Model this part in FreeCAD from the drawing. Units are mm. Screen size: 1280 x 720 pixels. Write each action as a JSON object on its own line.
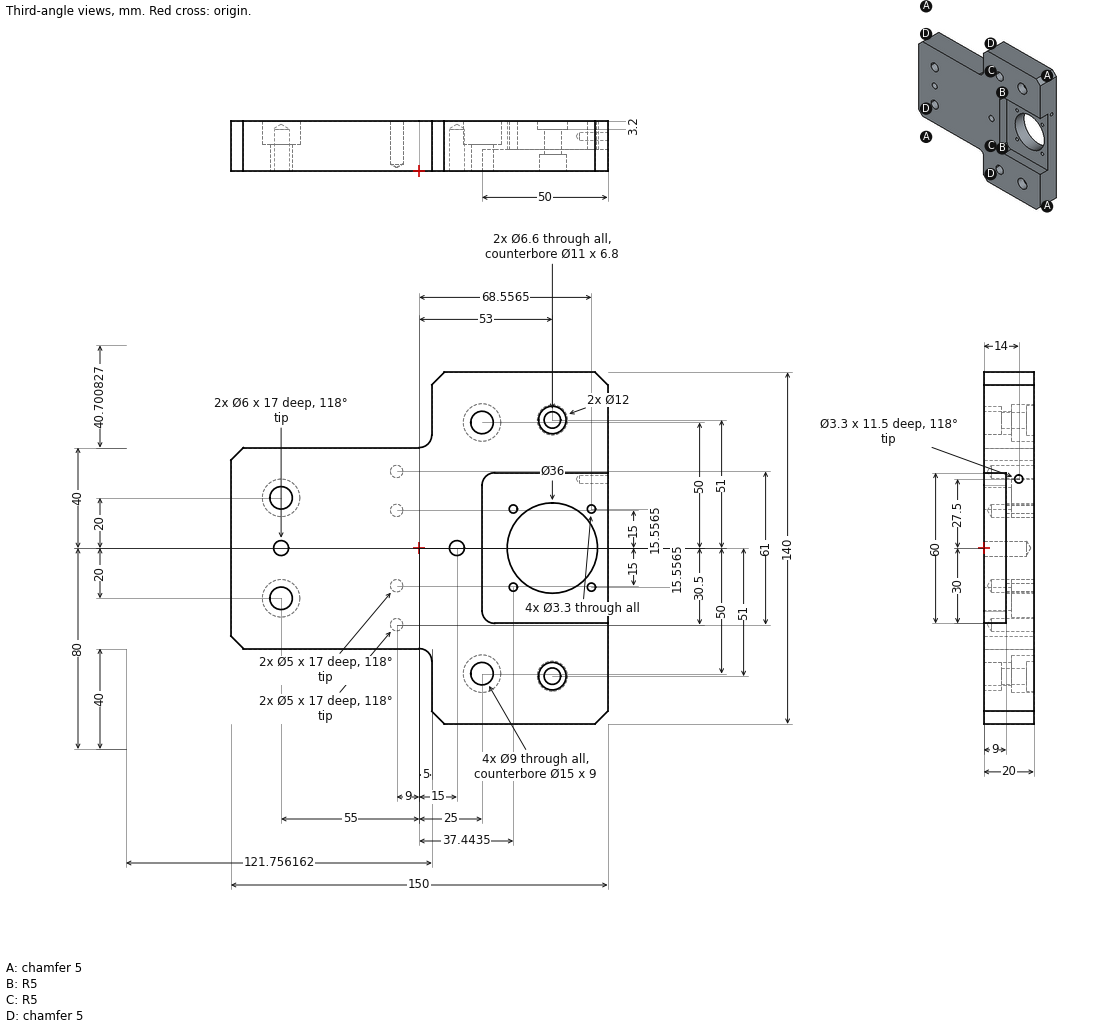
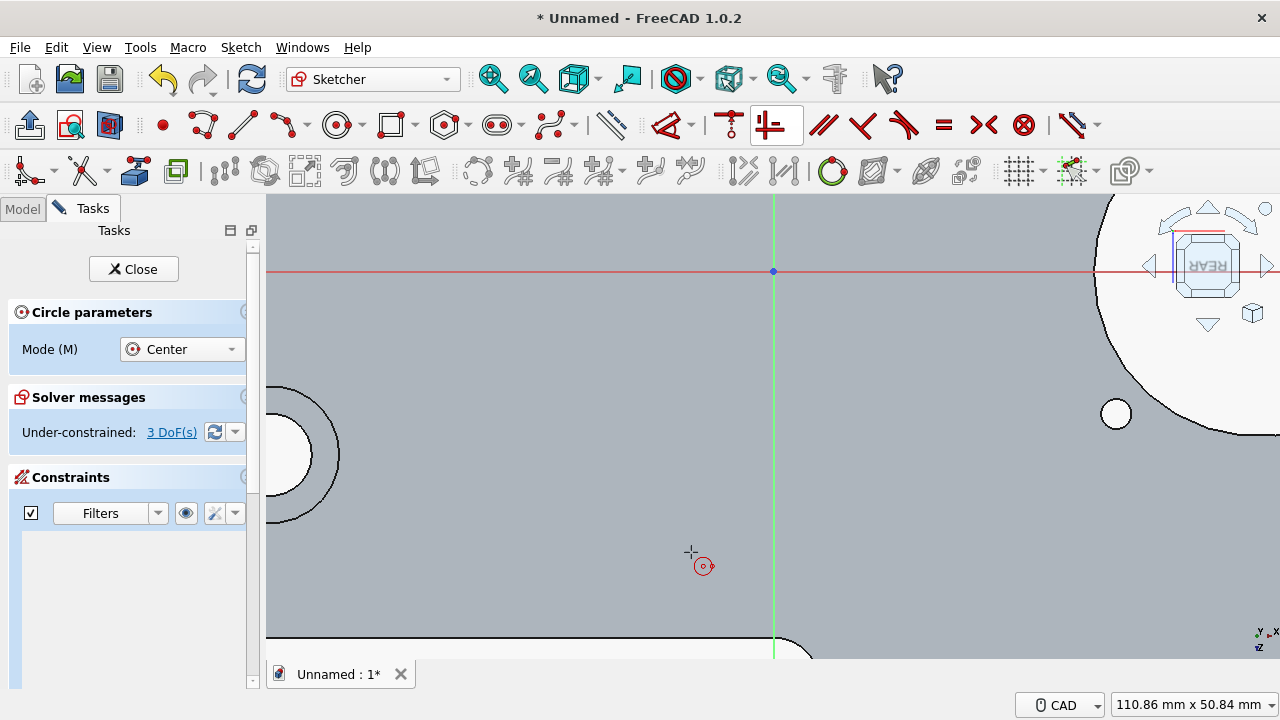
{"action": "left_click", "coordinate": [691, 551]}
{"action": "left_click", "coordinate": [708, 535]}
{"action": "key", "text": "Escape"}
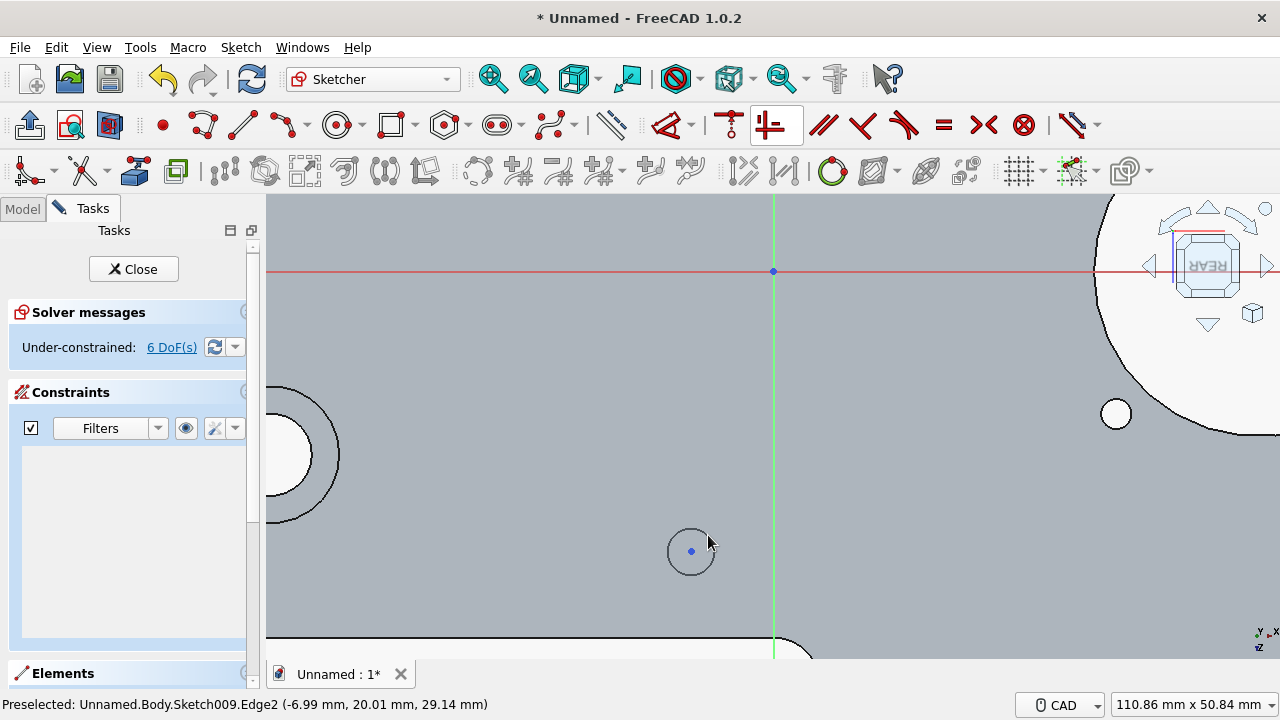
{"action": "scroll", "coordinate": [691, 553], "scroll_direction": "down", "scroll_amount": 4}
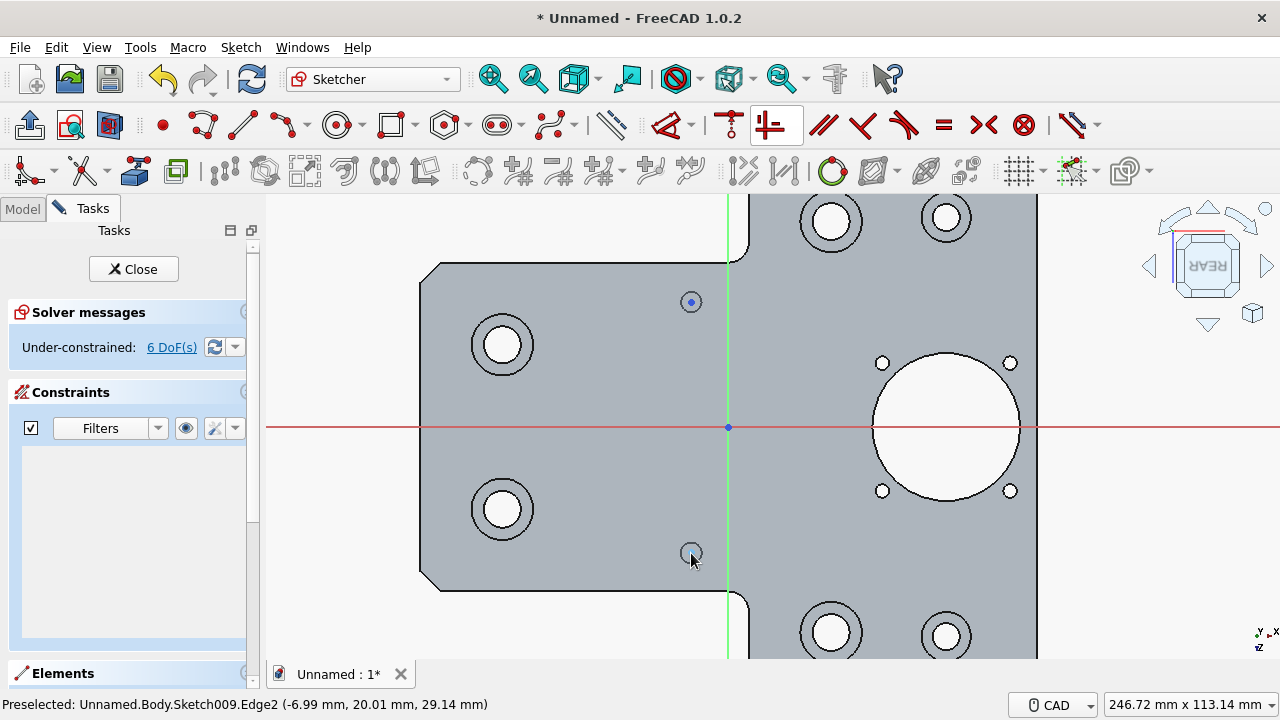
{"action": "scroll", "coordinate": [698, 295], "scroll_direction": "up", "scroll_amount": 2}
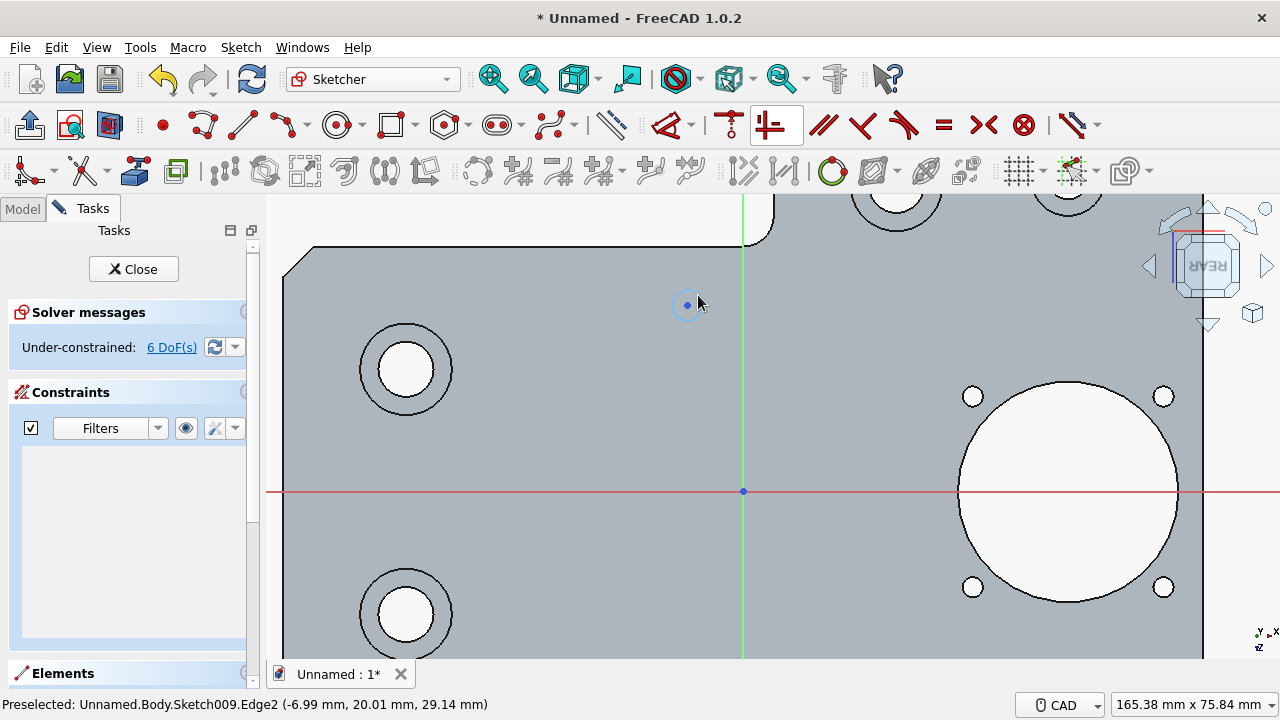
{"action": "left_click", "coordinate": [699, 295]}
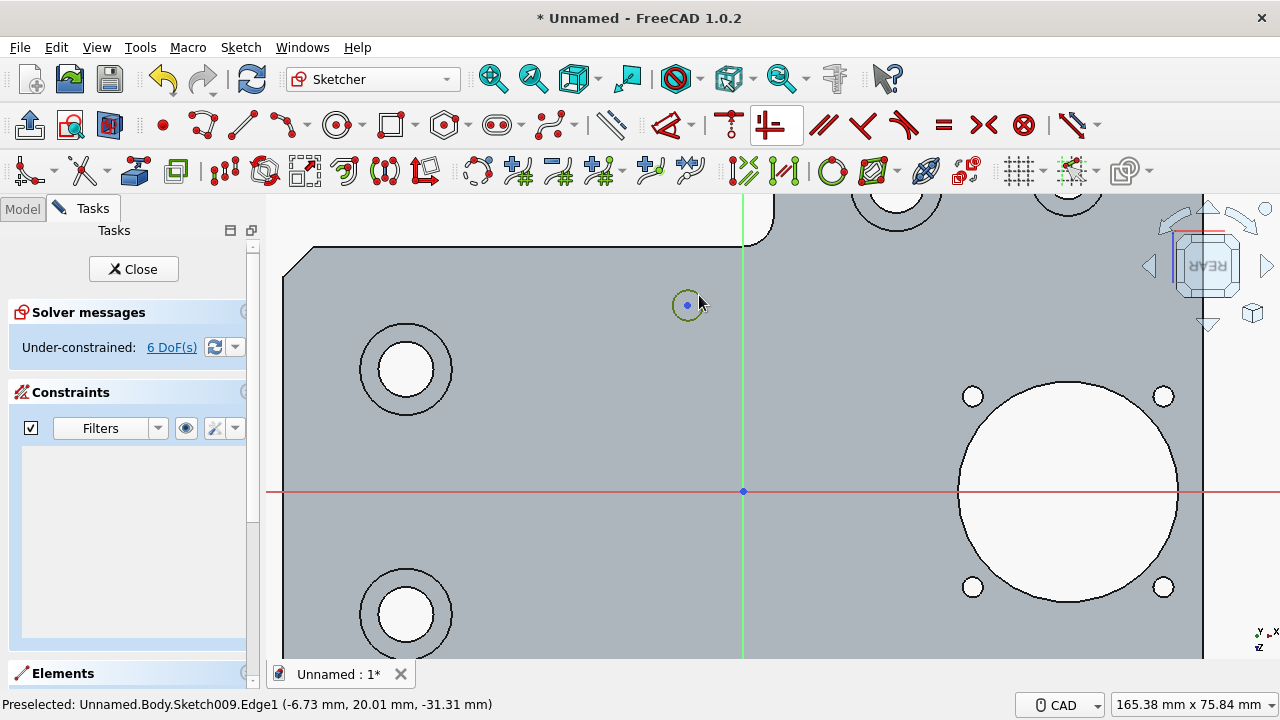
{"action": "scroll", "coordinate": [698, 294], "scroll_direction": "down", "scroll_amount": 2}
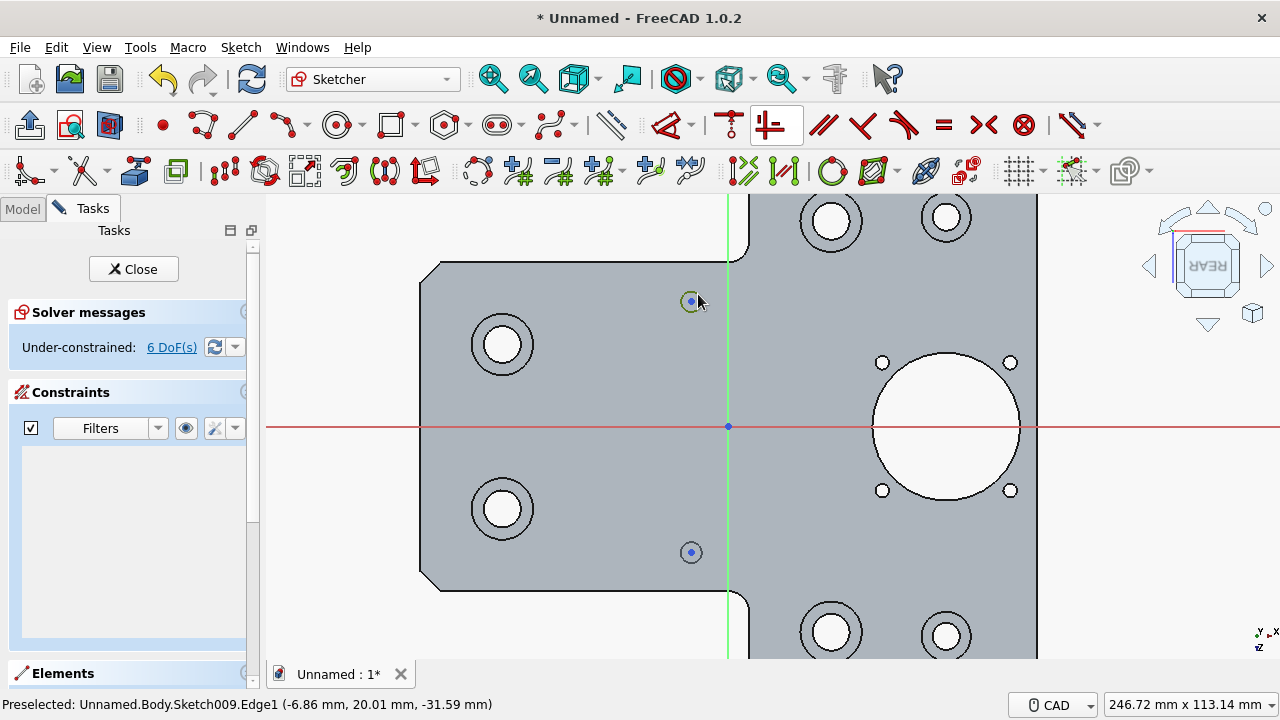
{"action": "scroll", "coordinate": [699, 545], "scroll_direction": "up", "scroll_amount": 2}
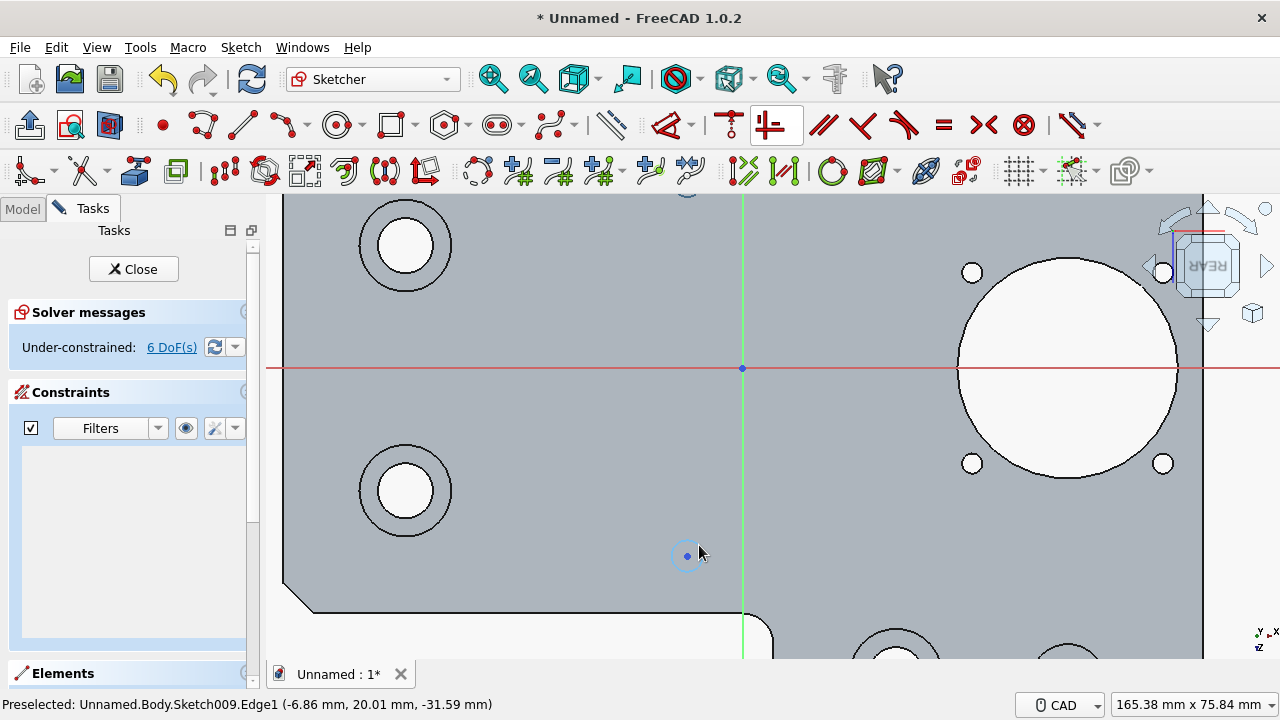
{"action": "left_click", "coordinate": [698, 545]}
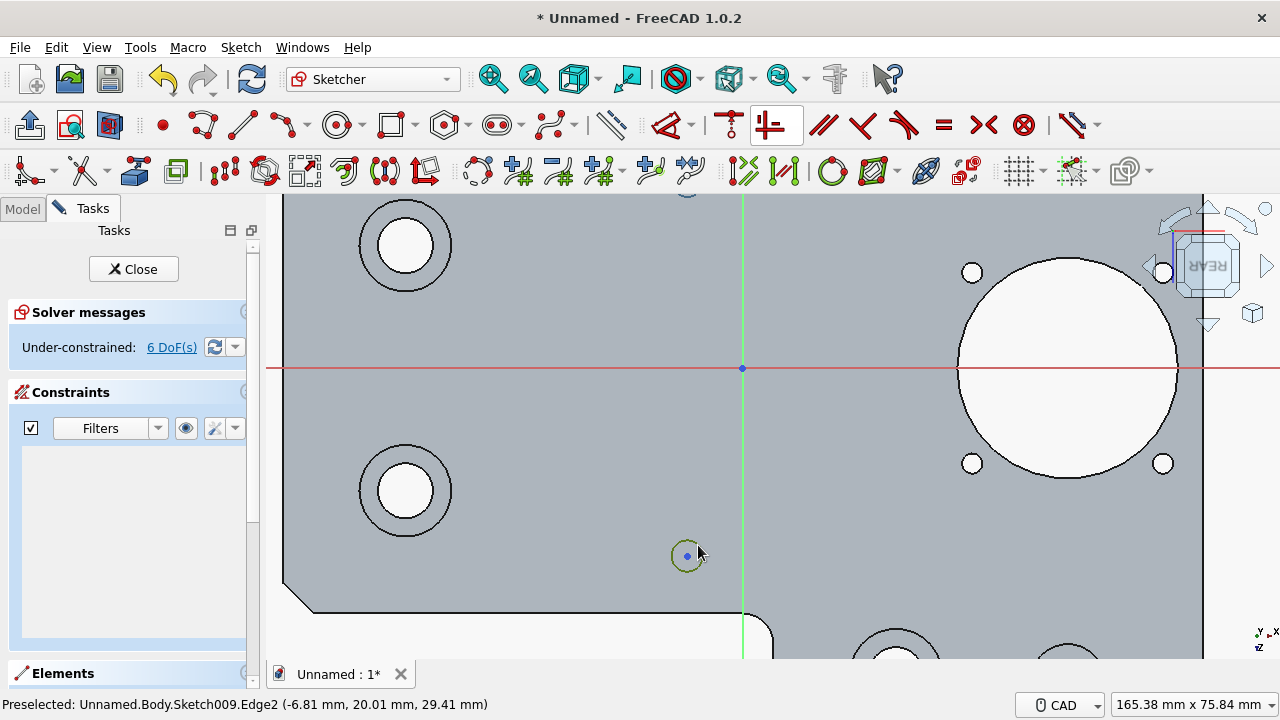
{"action": "left_click", "coordinate": [944, 126]}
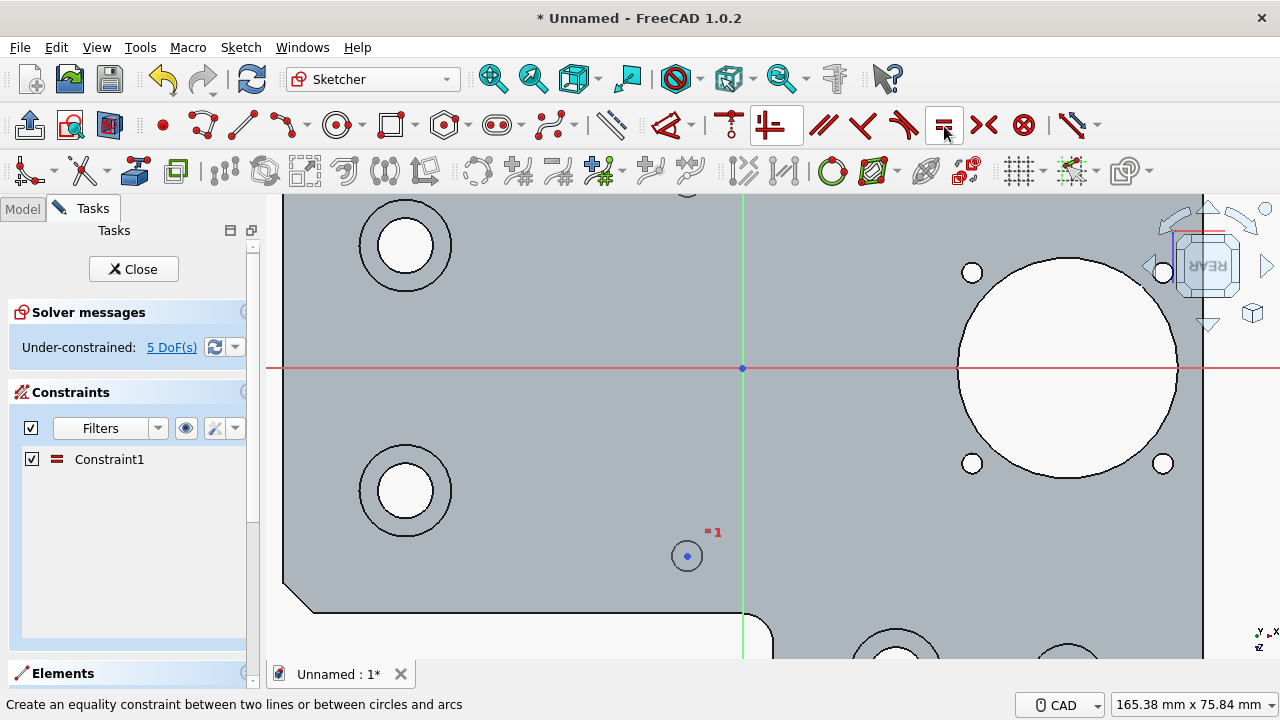
{"action": "scroll", "coordinate": [699, 545], "scroll_direction": "down", "scroll_amount": 2}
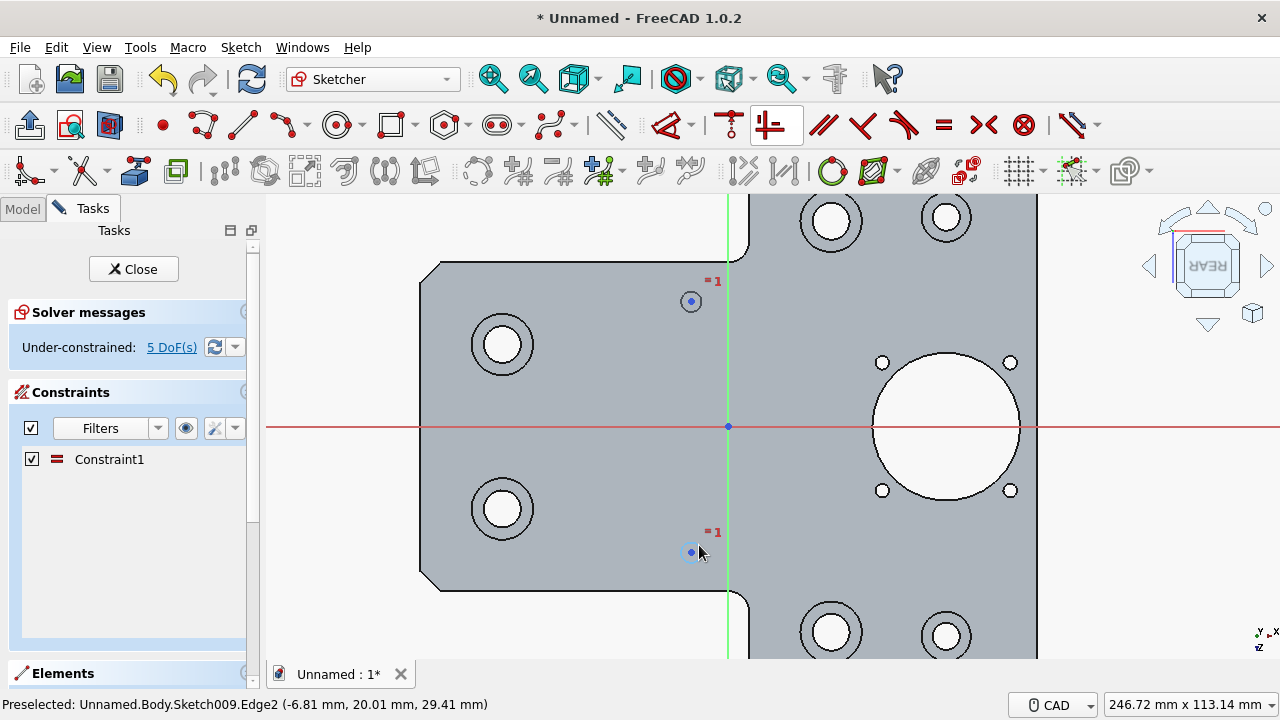
{"action": "left_click", "coordinate": [691, 302]}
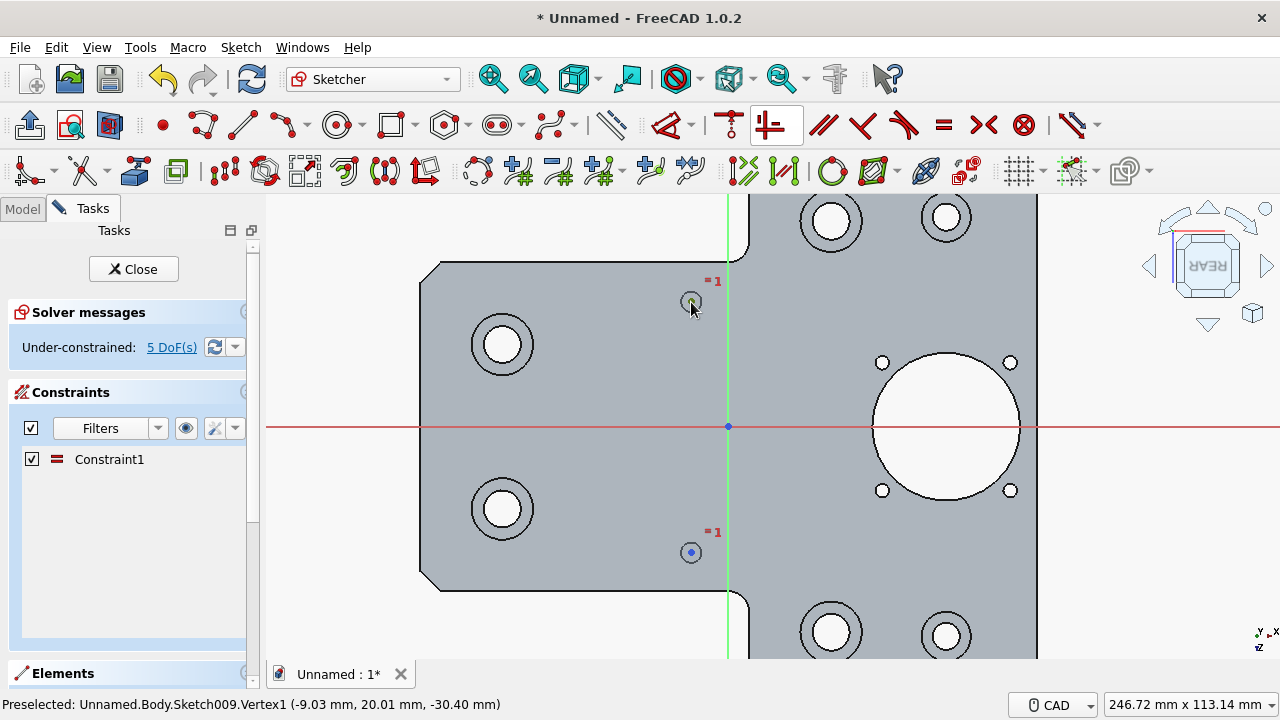
{"action": "left_click", "coordinate": [691, 553]}